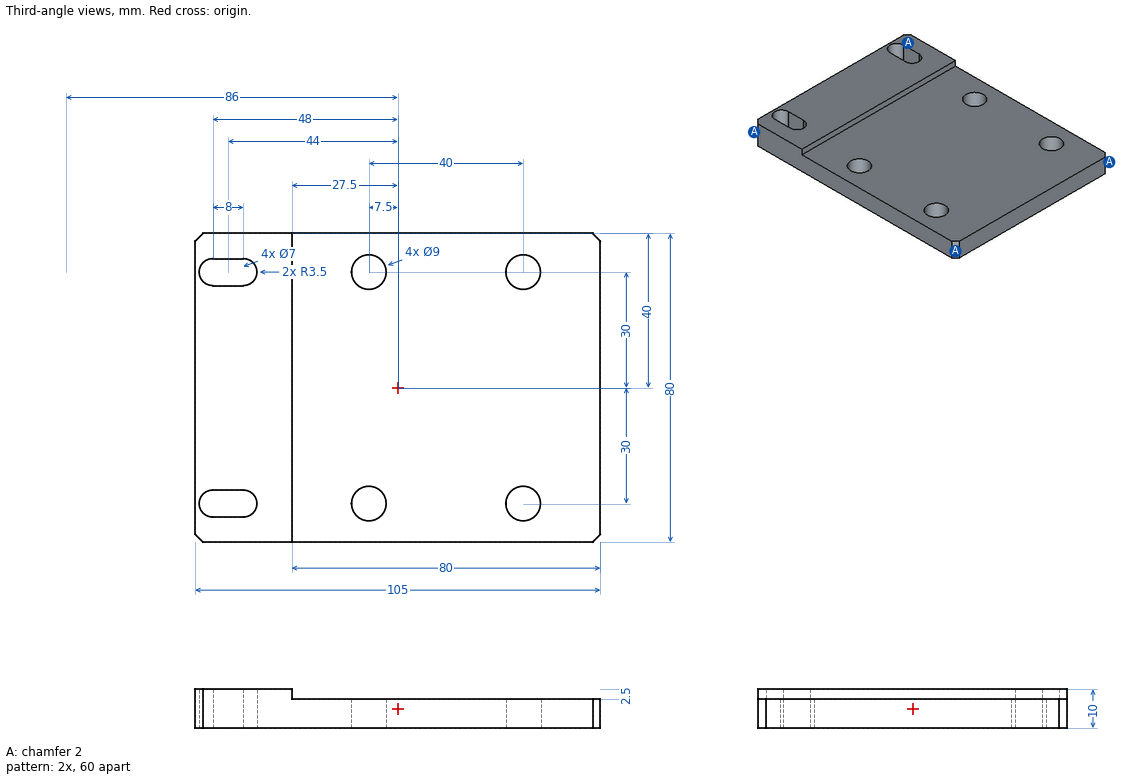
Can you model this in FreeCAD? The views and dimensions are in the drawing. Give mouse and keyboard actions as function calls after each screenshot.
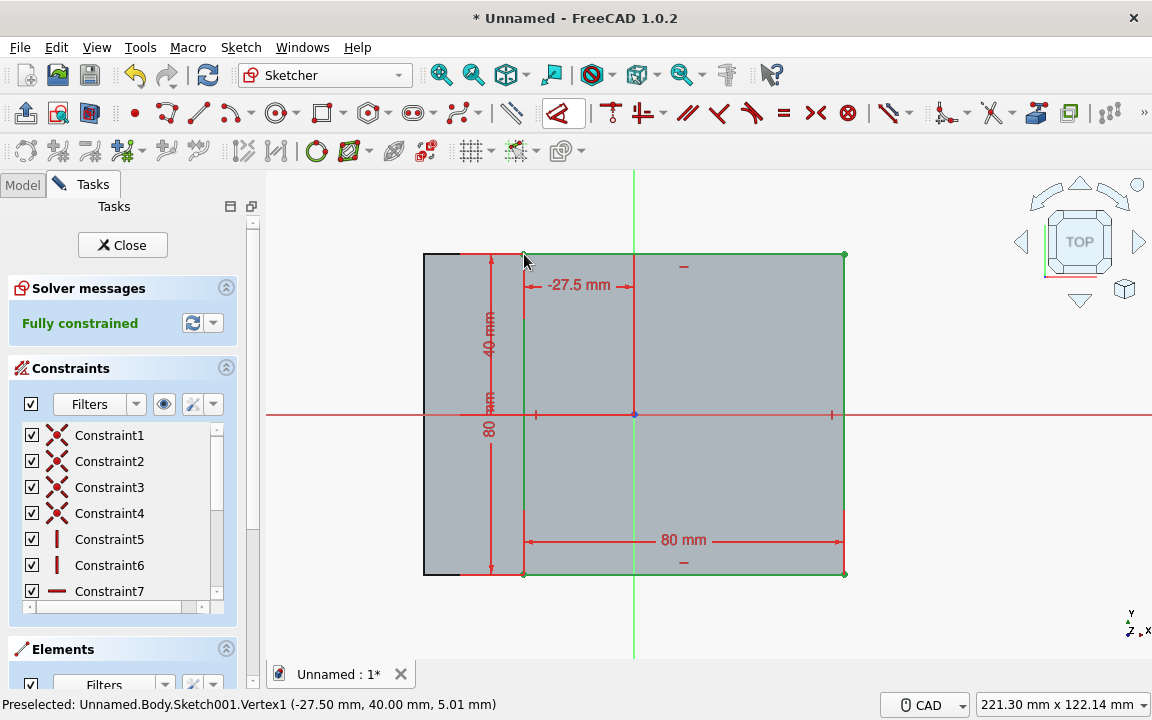
click(123, 245)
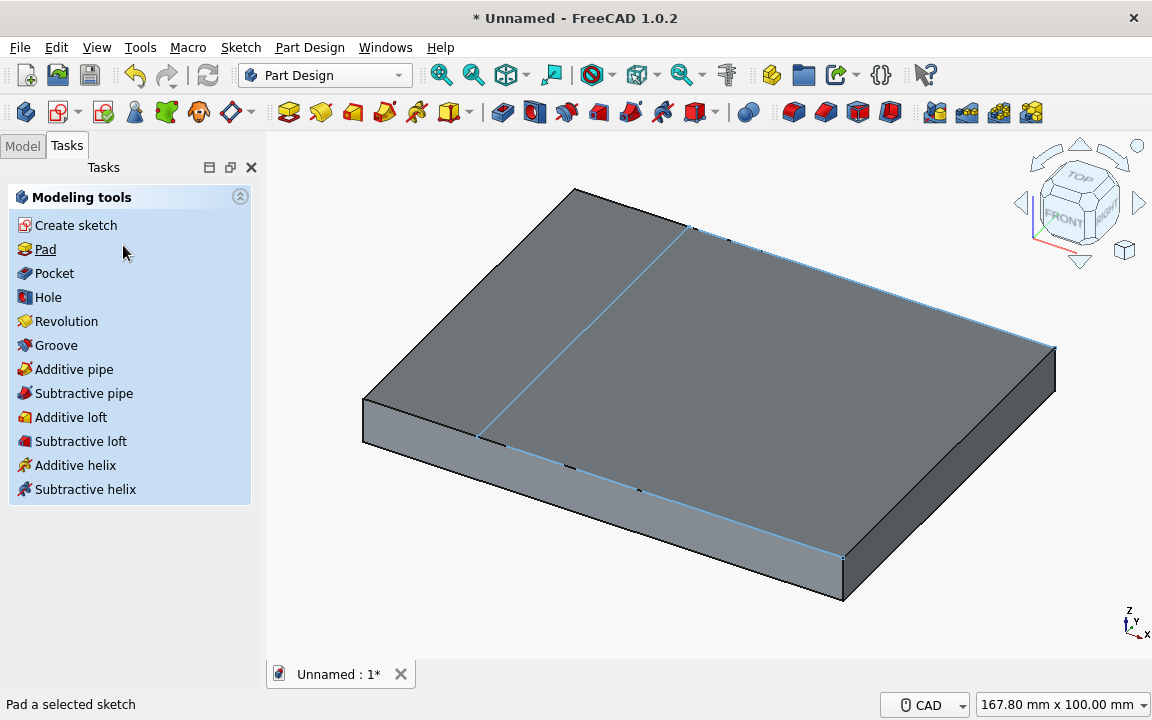
click(504, 112)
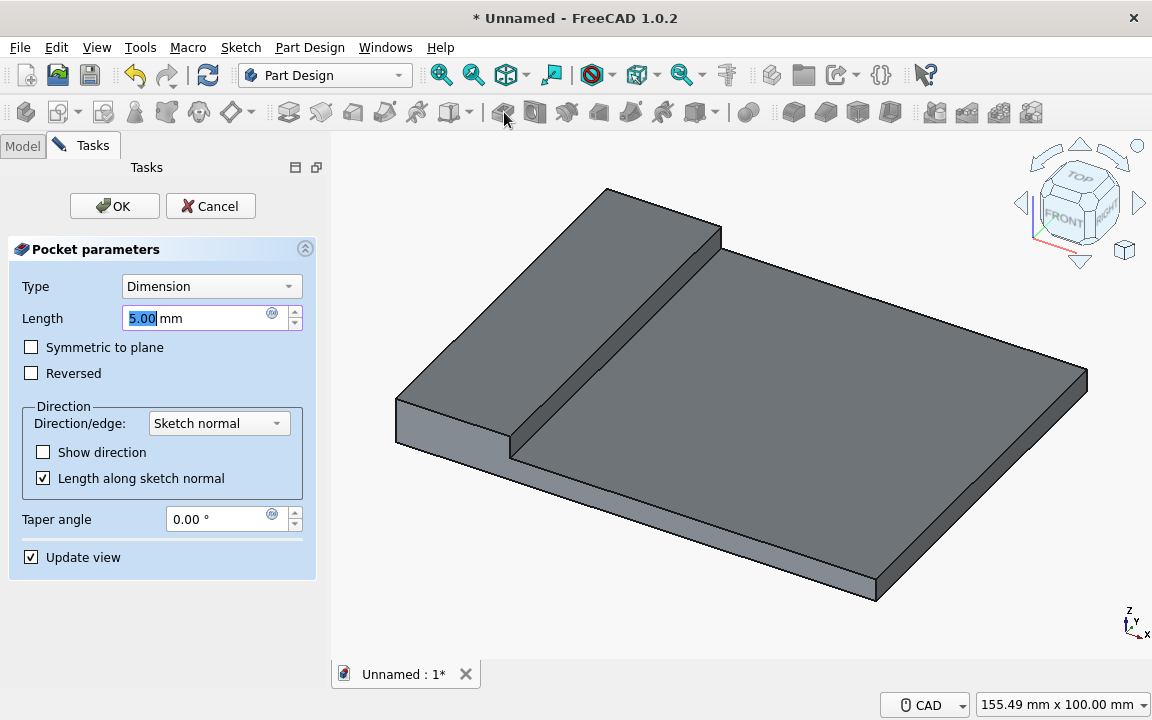
text(2.5)
key(Tab)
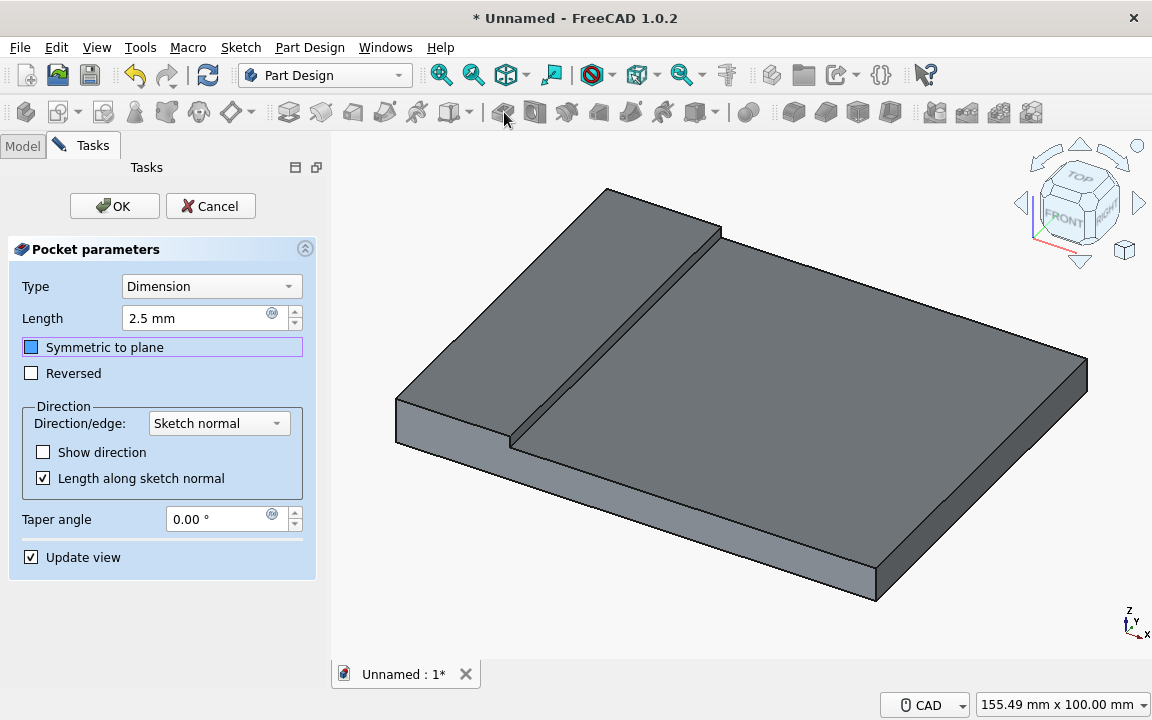
click(115, 206)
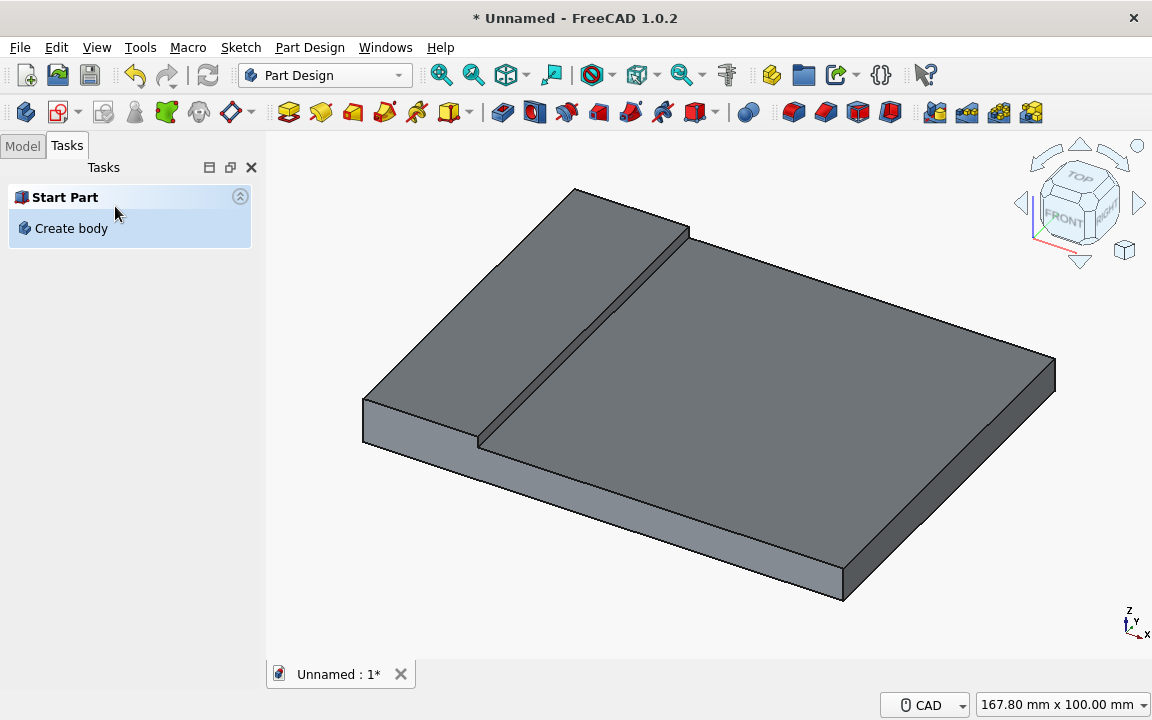
click(586, 252)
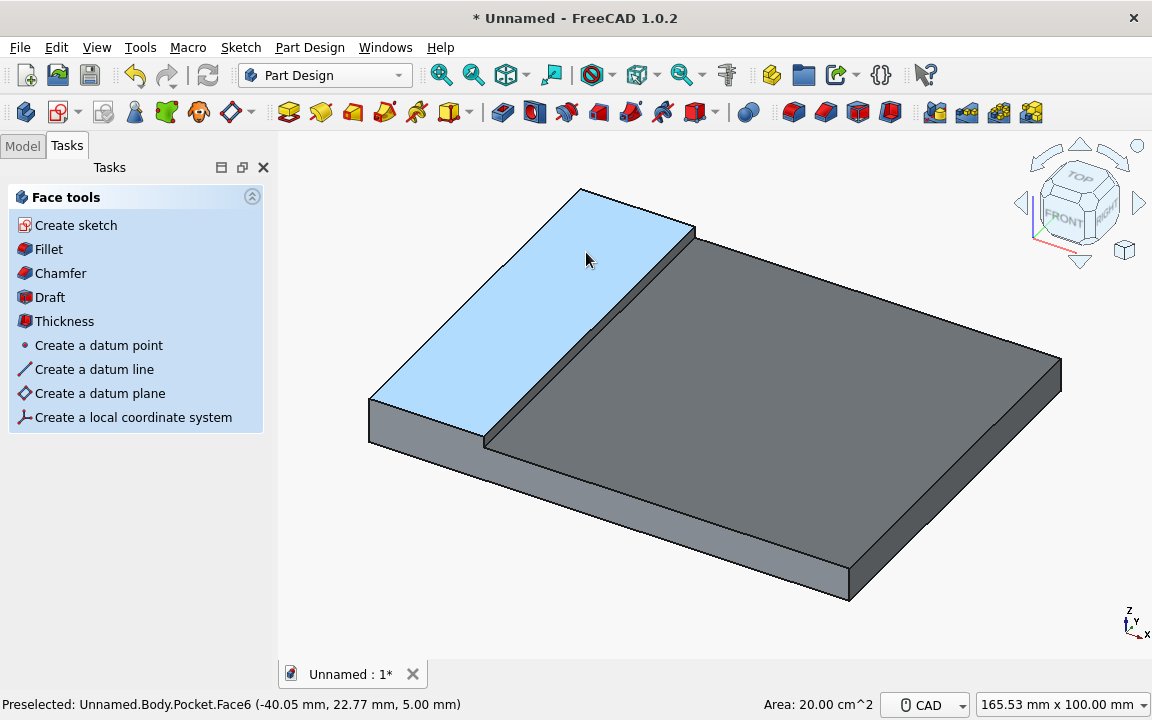
click(58, 112)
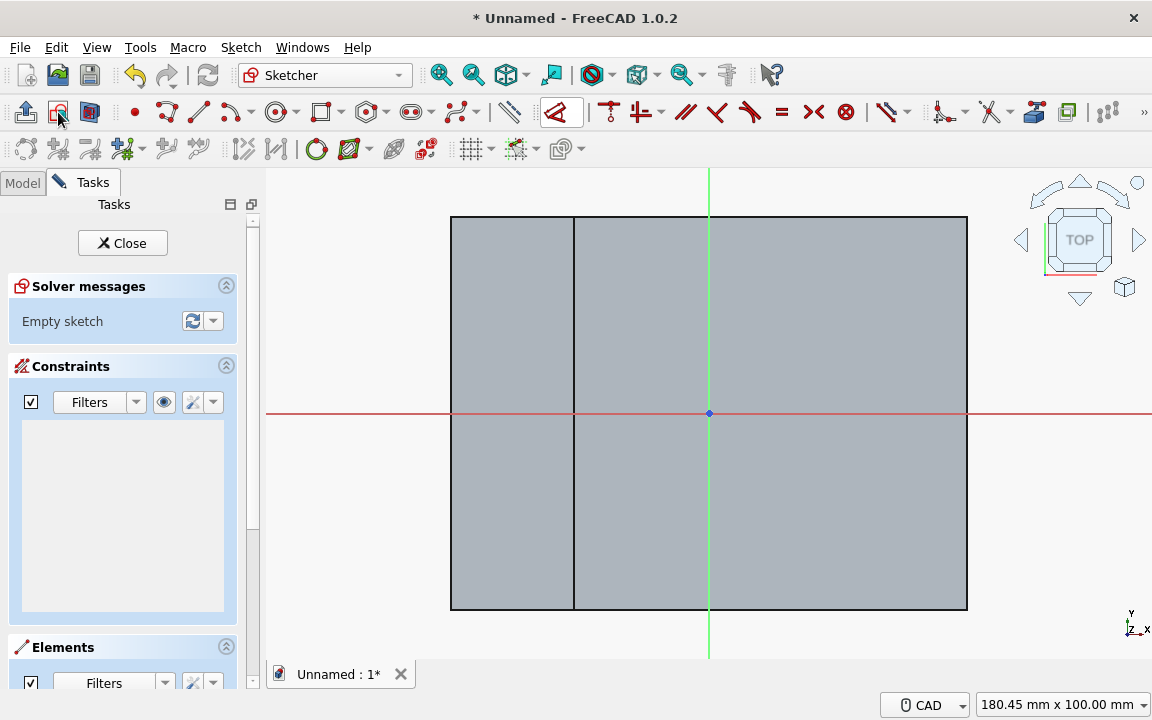
click(276, 112)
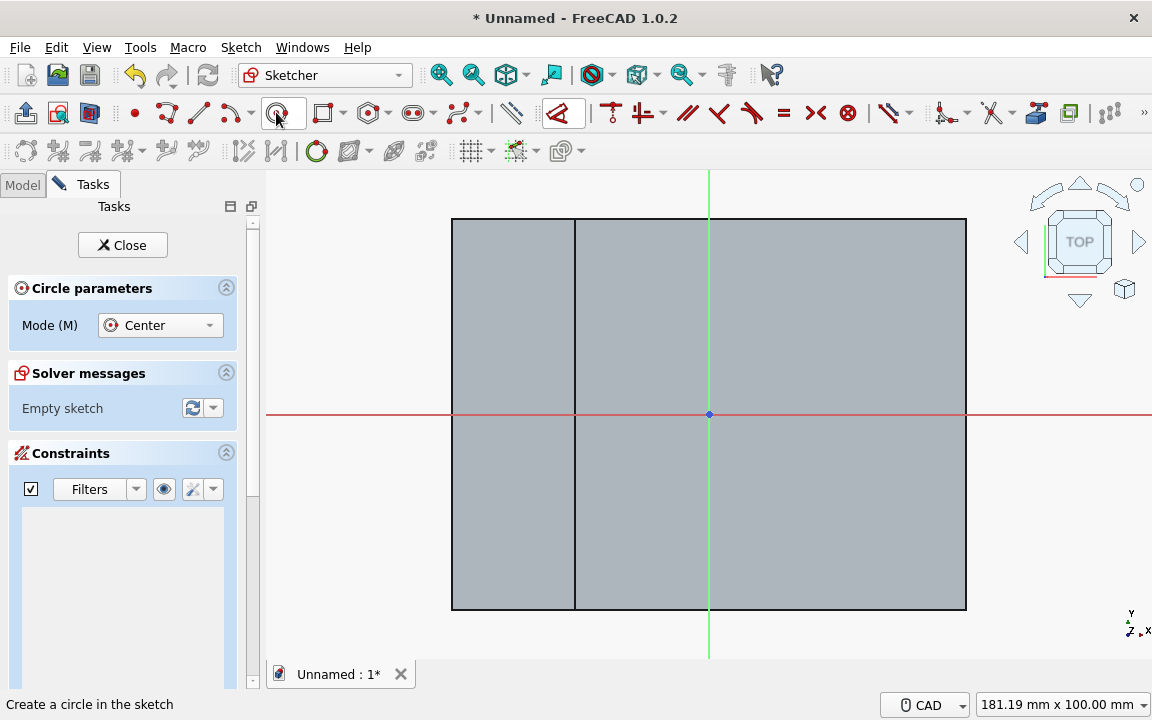
click(672, 268)
click(688, 252)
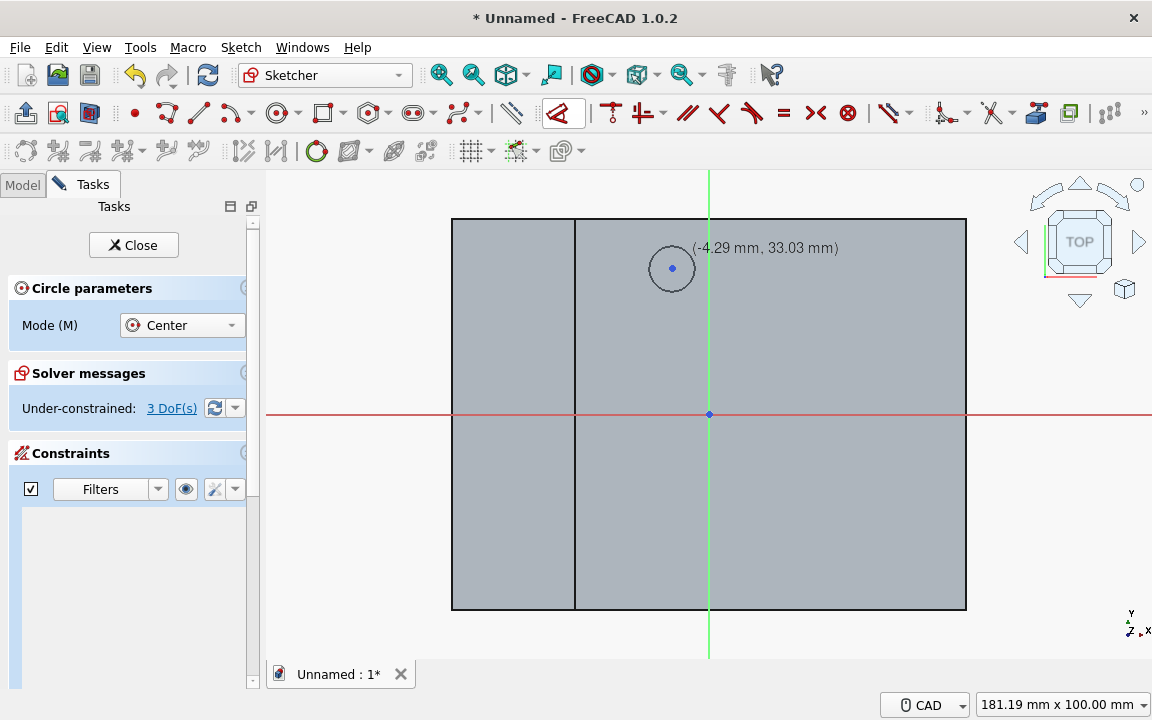
click(868, 268)
click(883, 252)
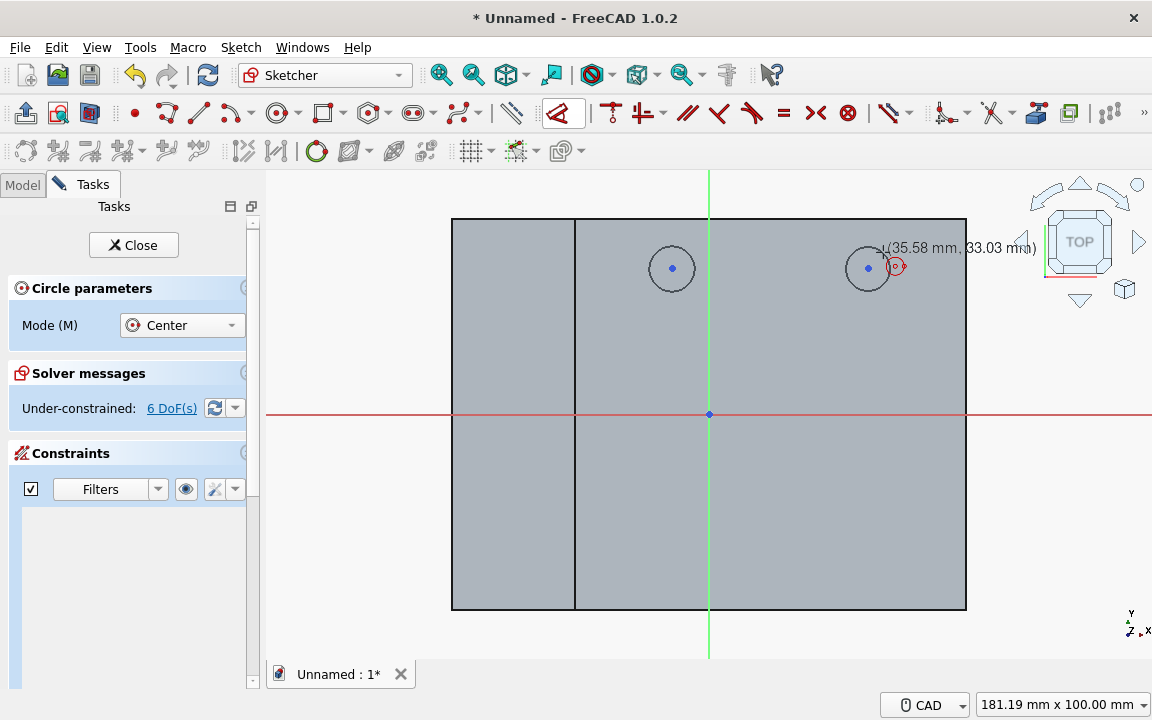
click(868, 561)
click(883, 546)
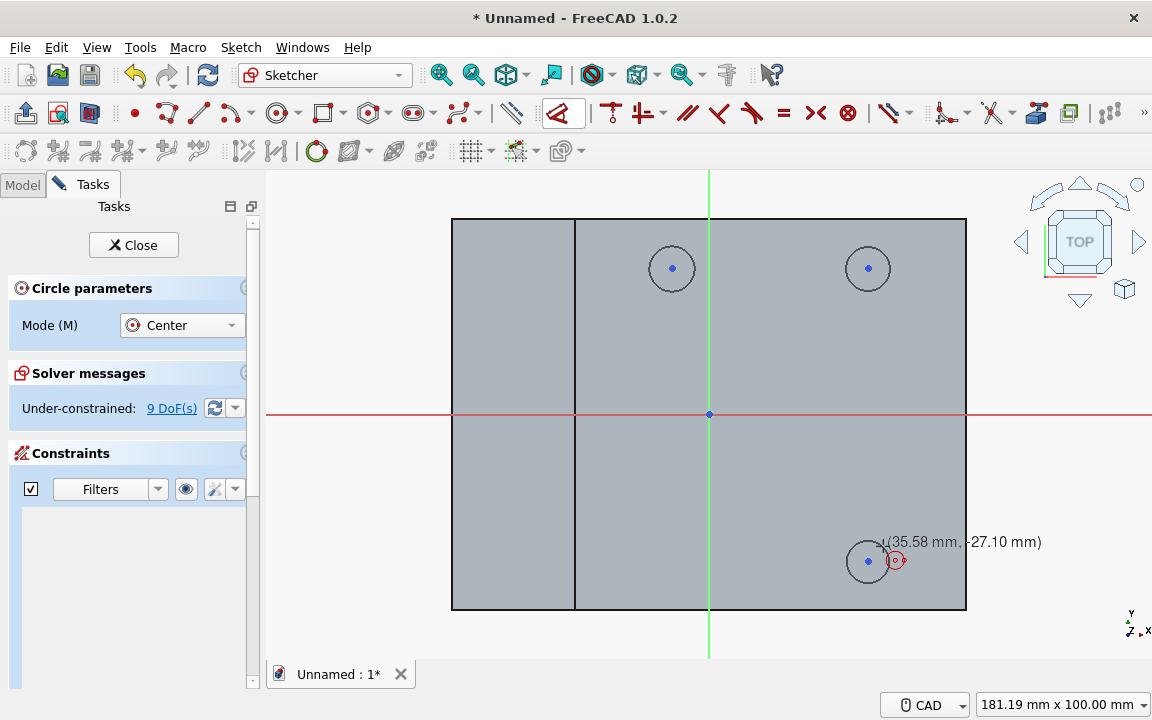
click(672, 561)
click(688, 546)
key(Escape)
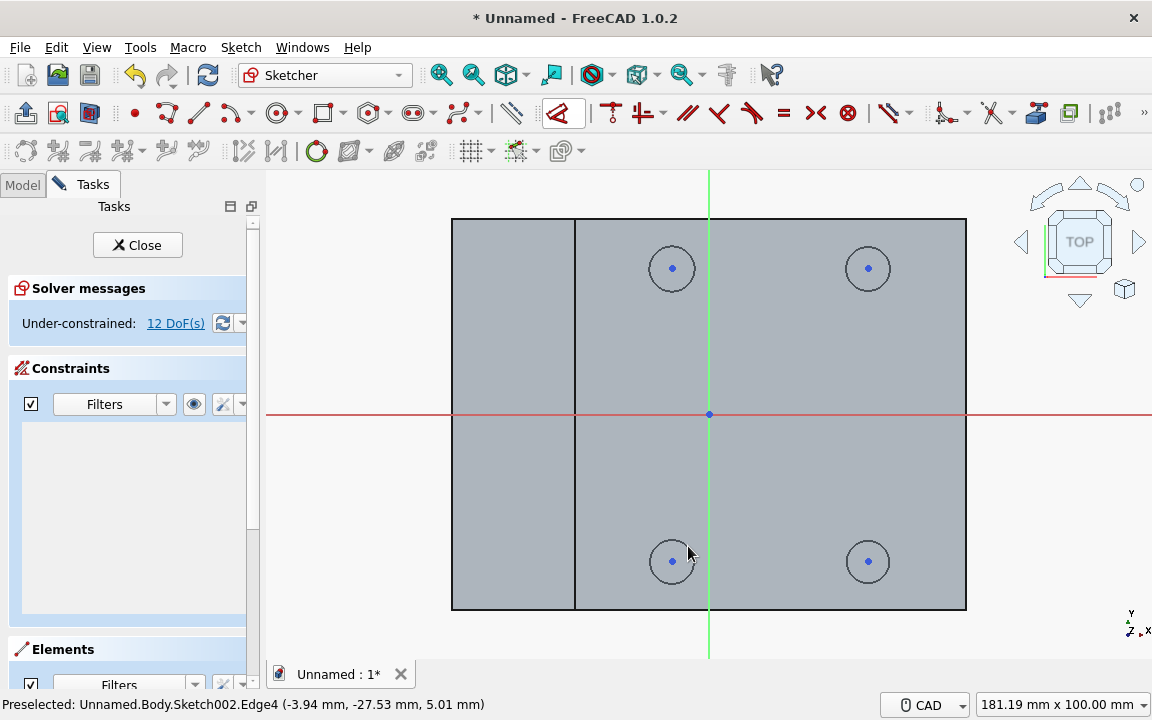
click(688, 253)